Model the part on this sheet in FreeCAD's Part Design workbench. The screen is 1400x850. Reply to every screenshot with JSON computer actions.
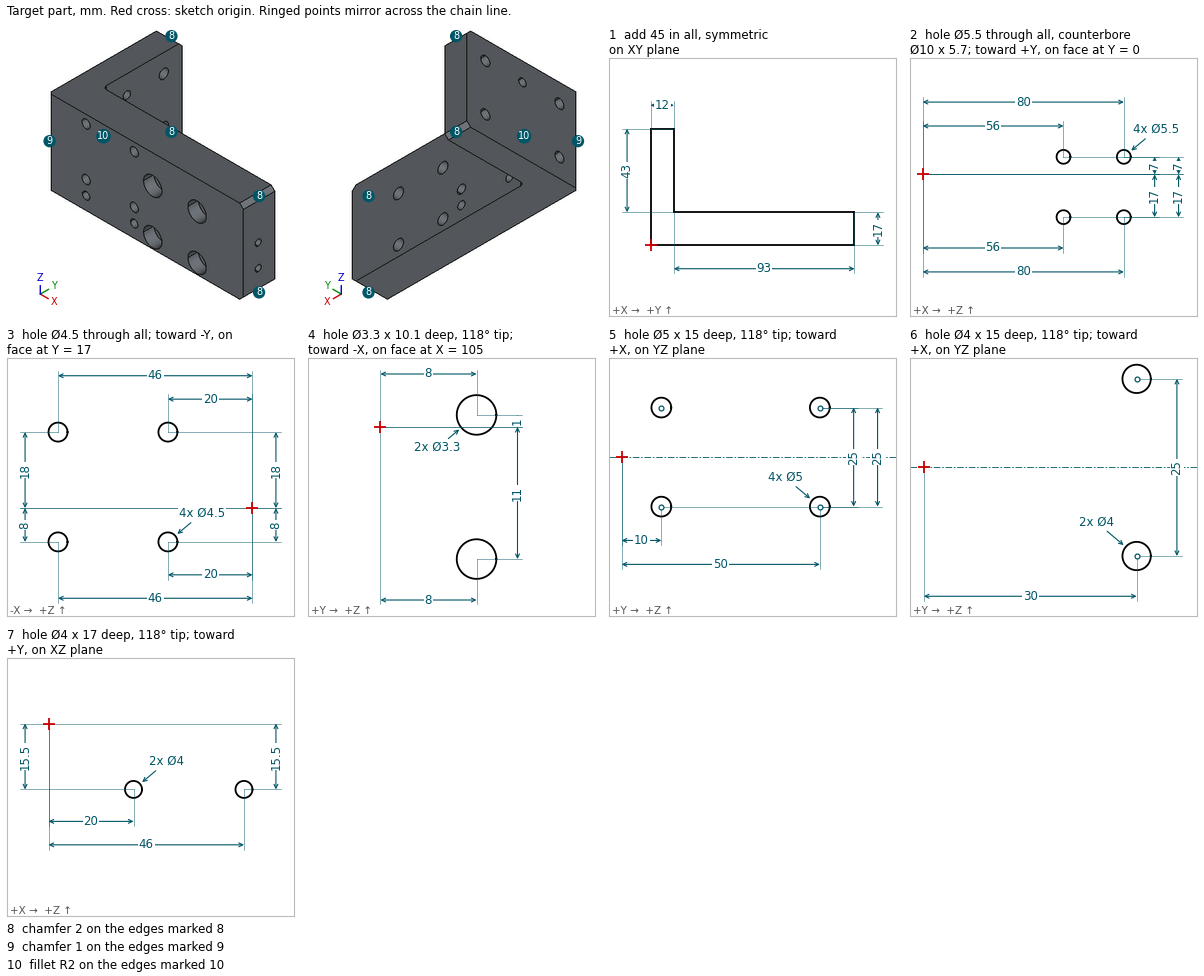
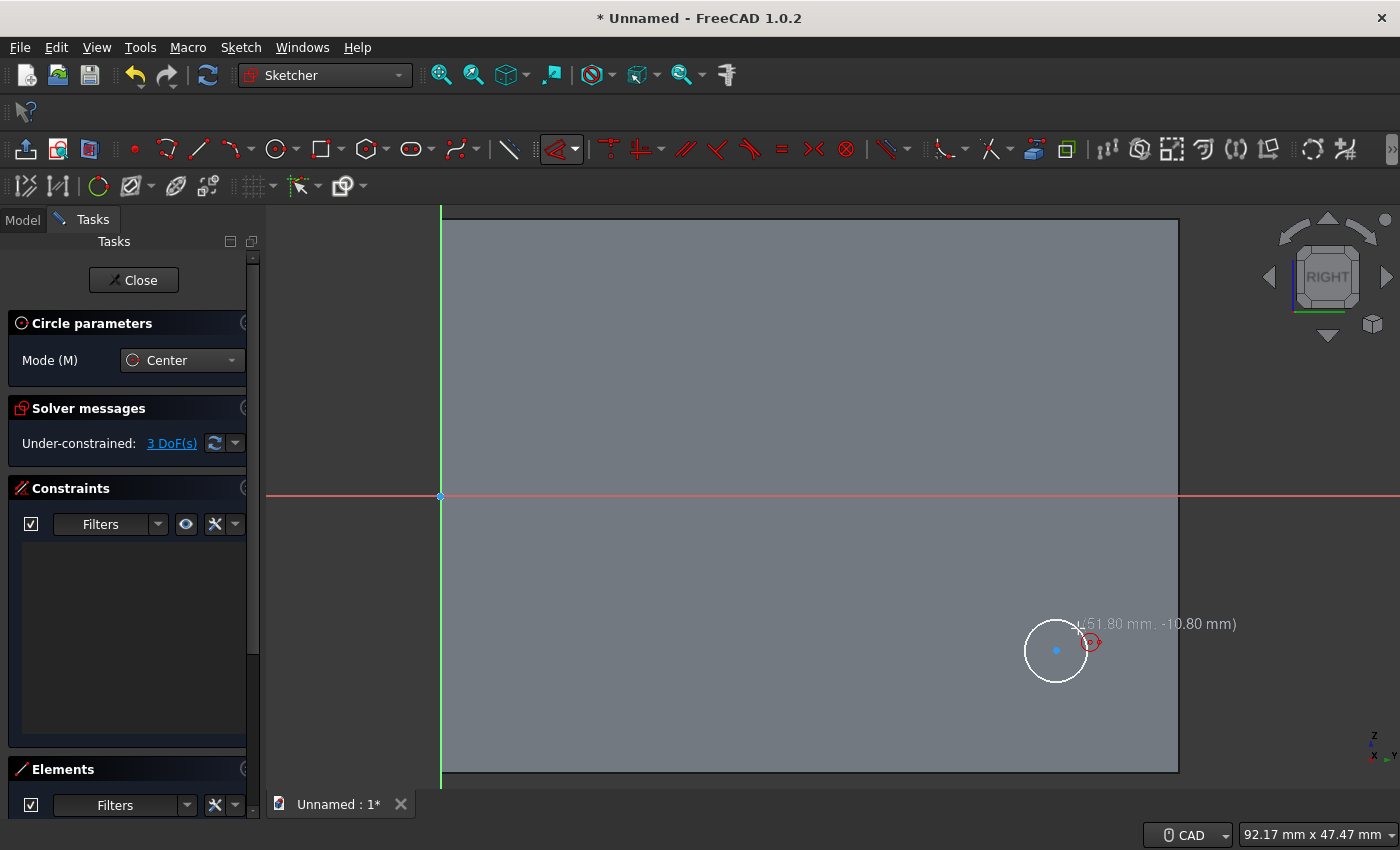
{"action": "left_click", "coordinate": [1056, 342]}
{"action": "left_click", "coordinate": [1078, 321]}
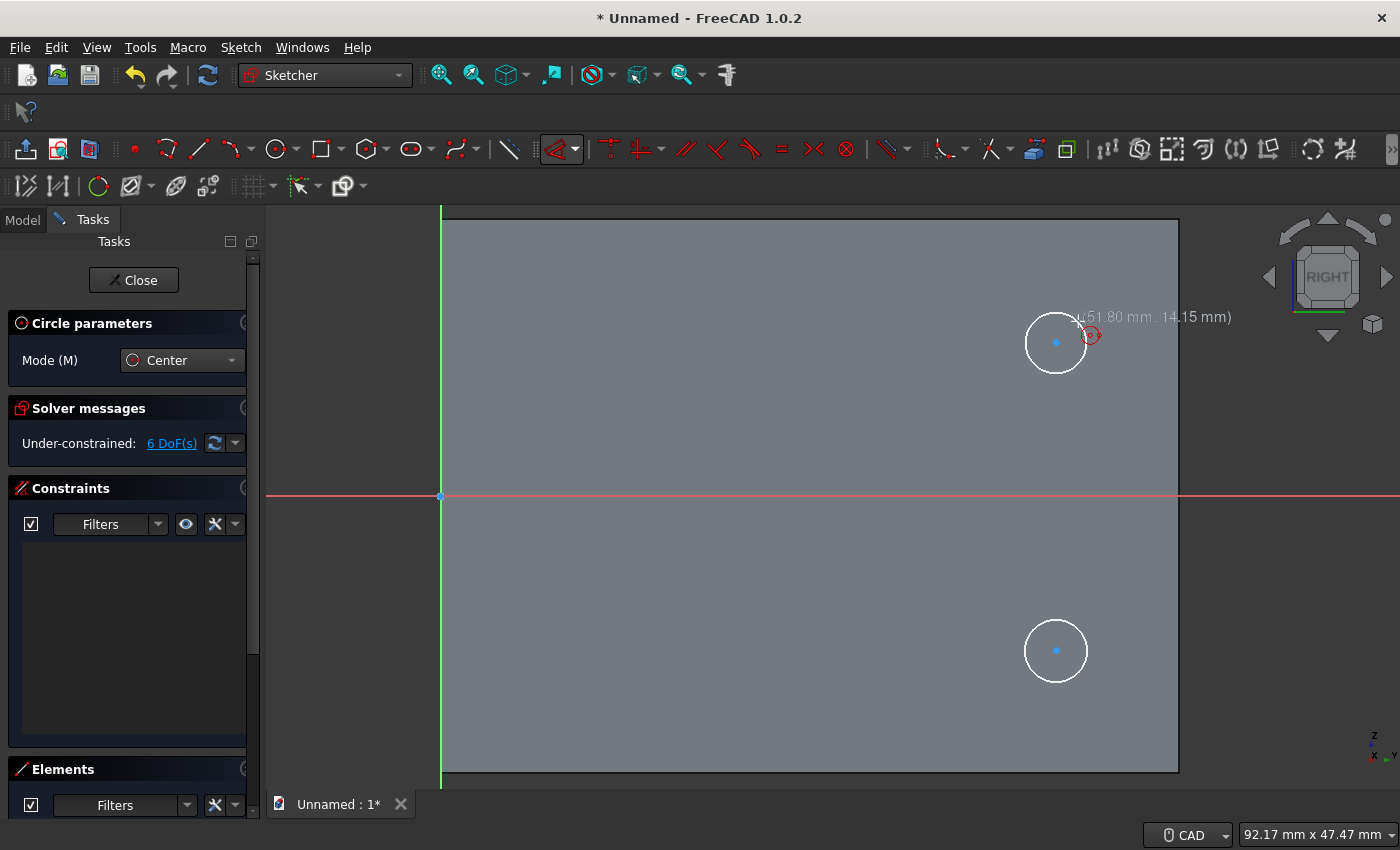
{"action": "left_click", "coordinate": [564, 650]}
{"action": "left_click", "coordinate": [585, 628]}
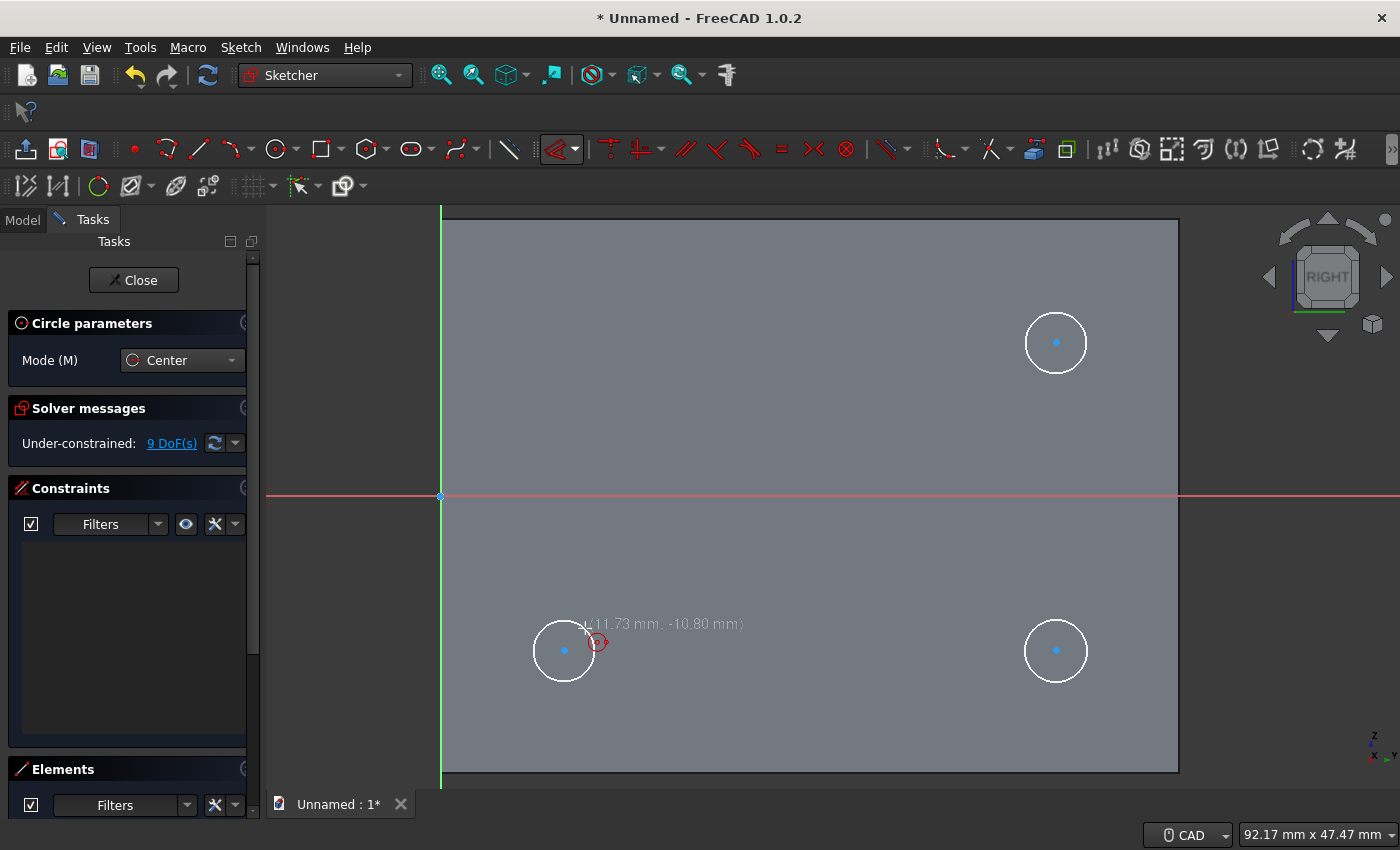
{"action": "left_click", "coordinate": [564, 342]}
{"action": "left_click", "coordinate": [585, 321]}
{"action": "key", "text": "Escape"}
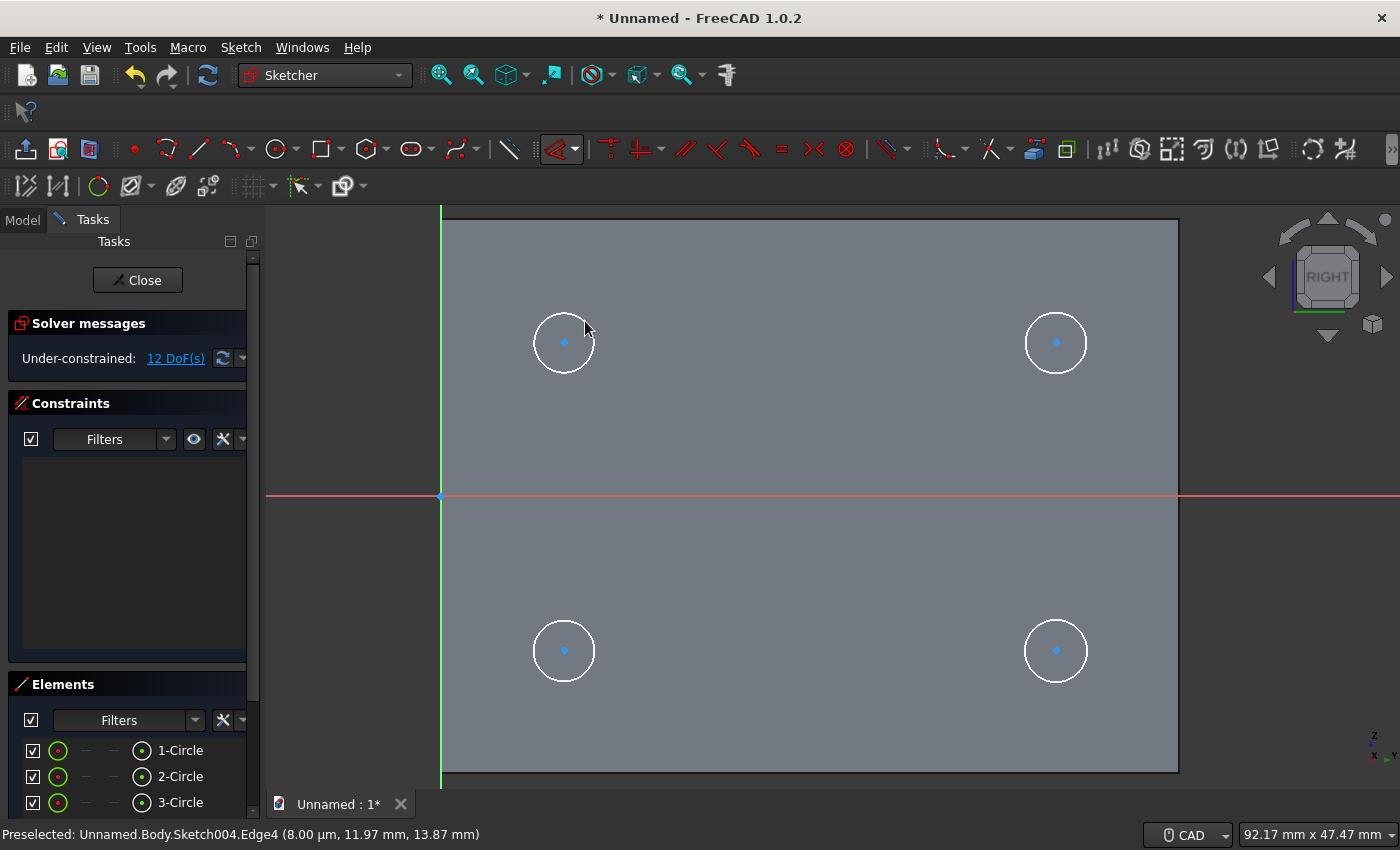
{"action": "left_click", "coordinate": [1078, 629]}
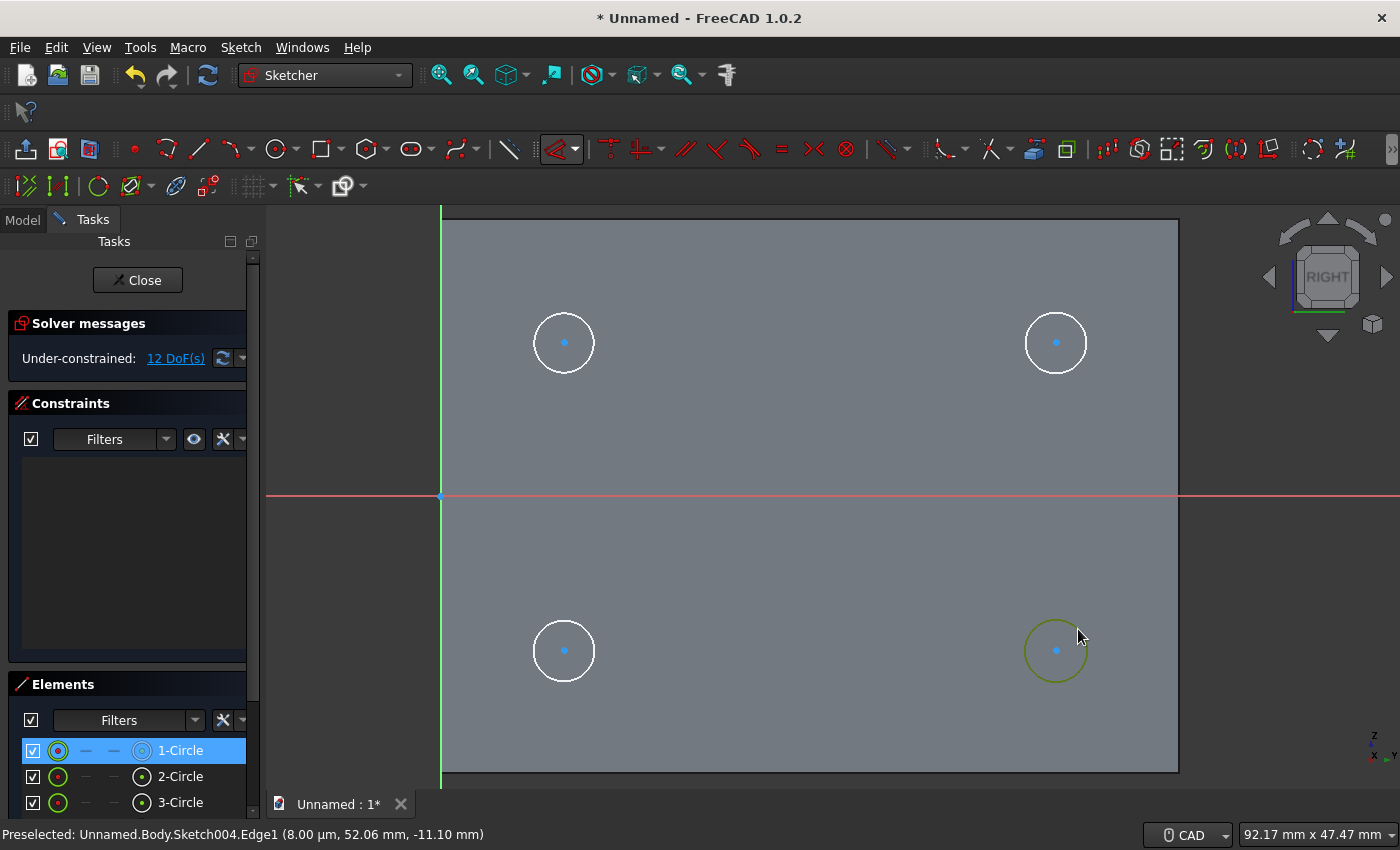
{"action": "left_click", "coordinate": [1077, 321]}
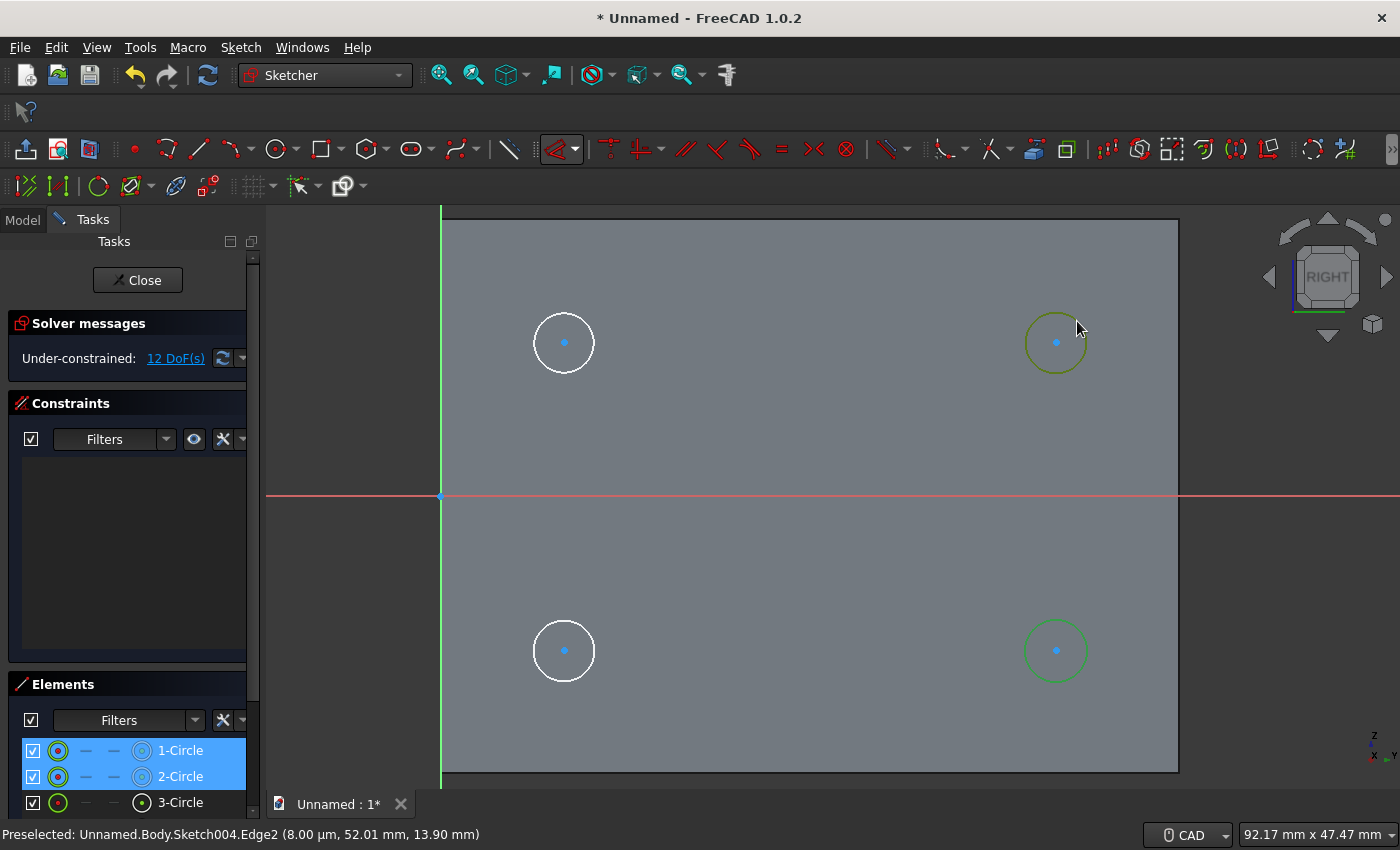
{"action": "left_click", "coordinate": [585, 629]}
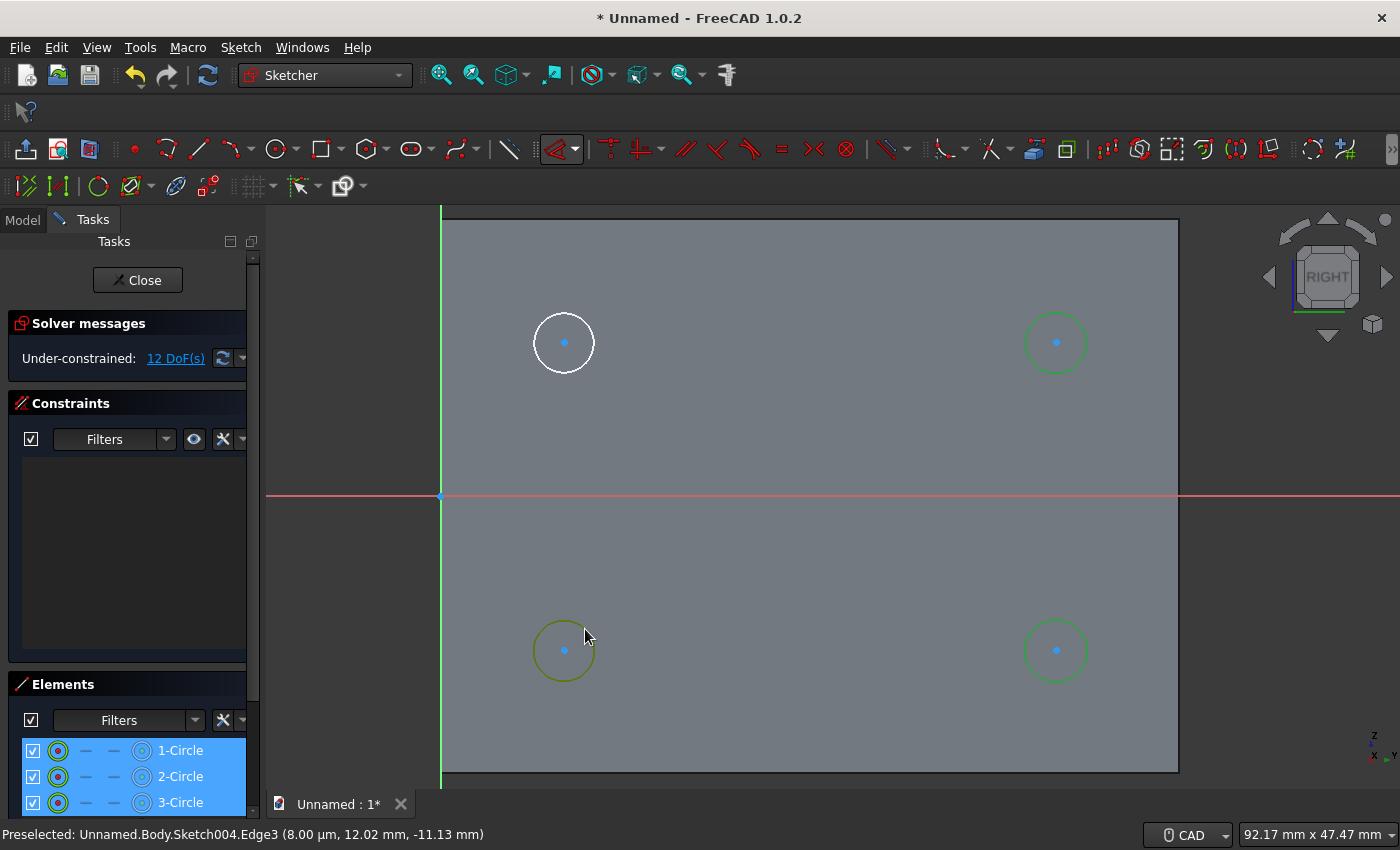
{"action": "left_click", "coordinate": [585, 322]}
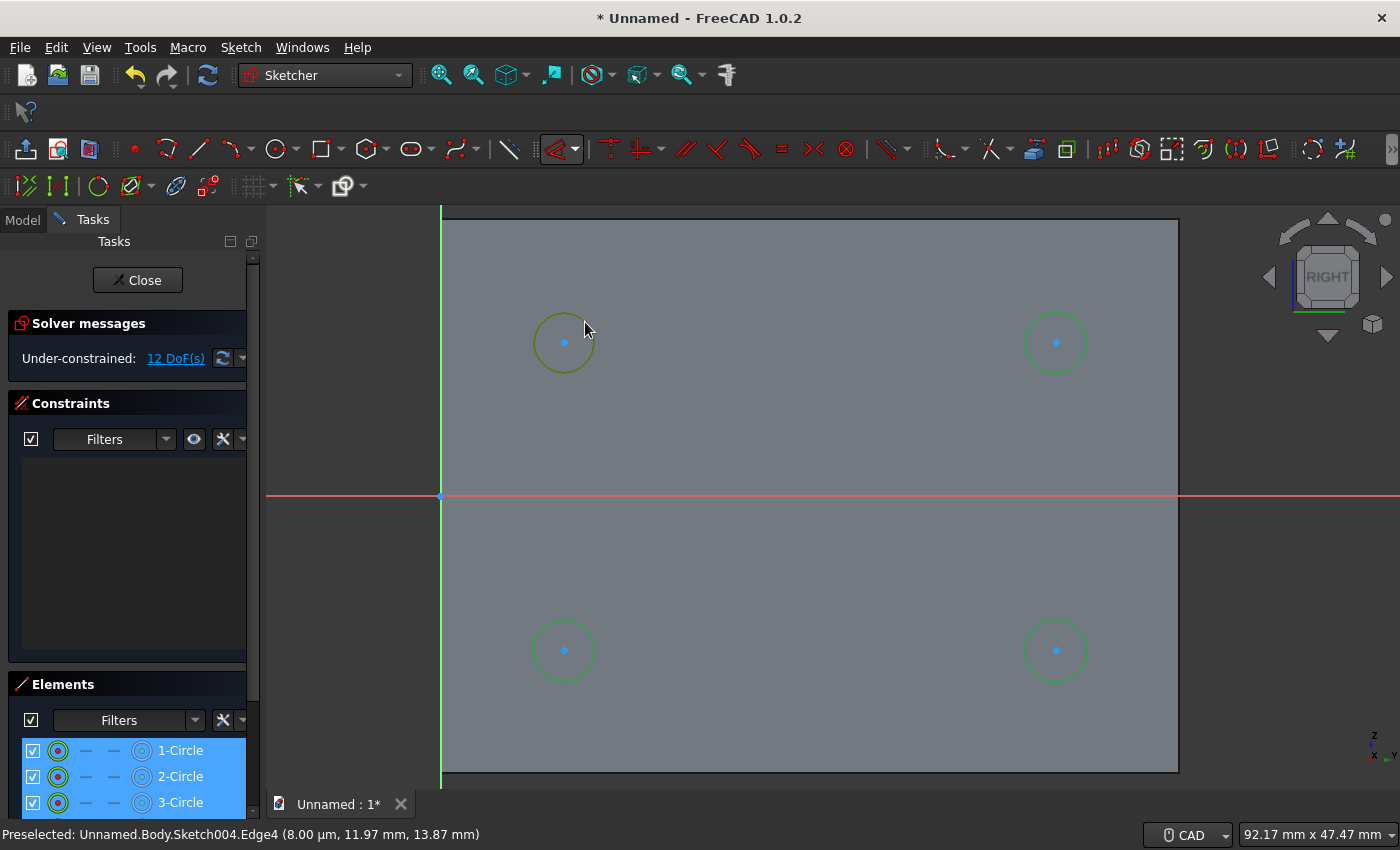
{"action": "key", "text": "e"}